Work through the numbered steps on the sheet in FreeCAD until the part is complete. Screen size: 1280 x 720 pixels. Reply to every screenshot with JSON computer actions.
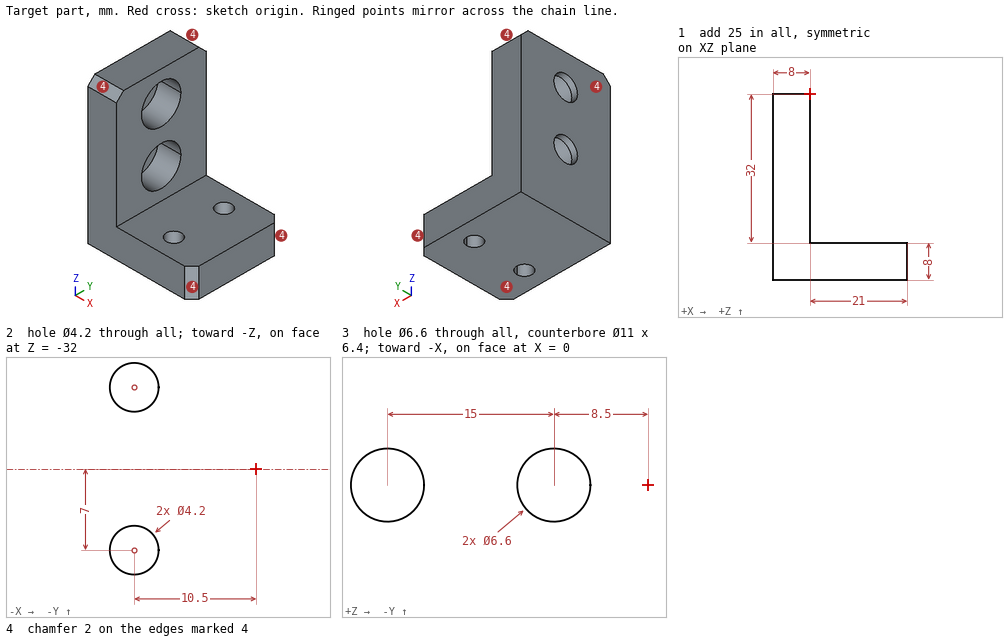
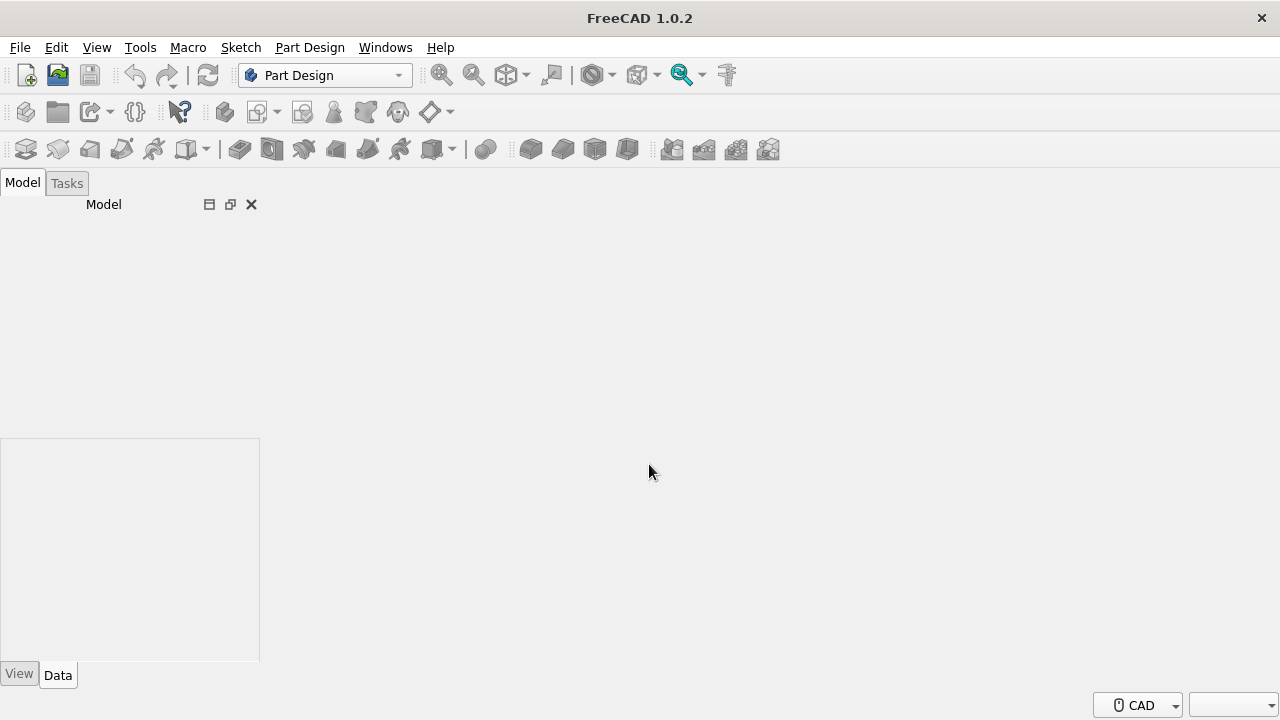
{"action": "left_click", "coordinate": [26, 76]}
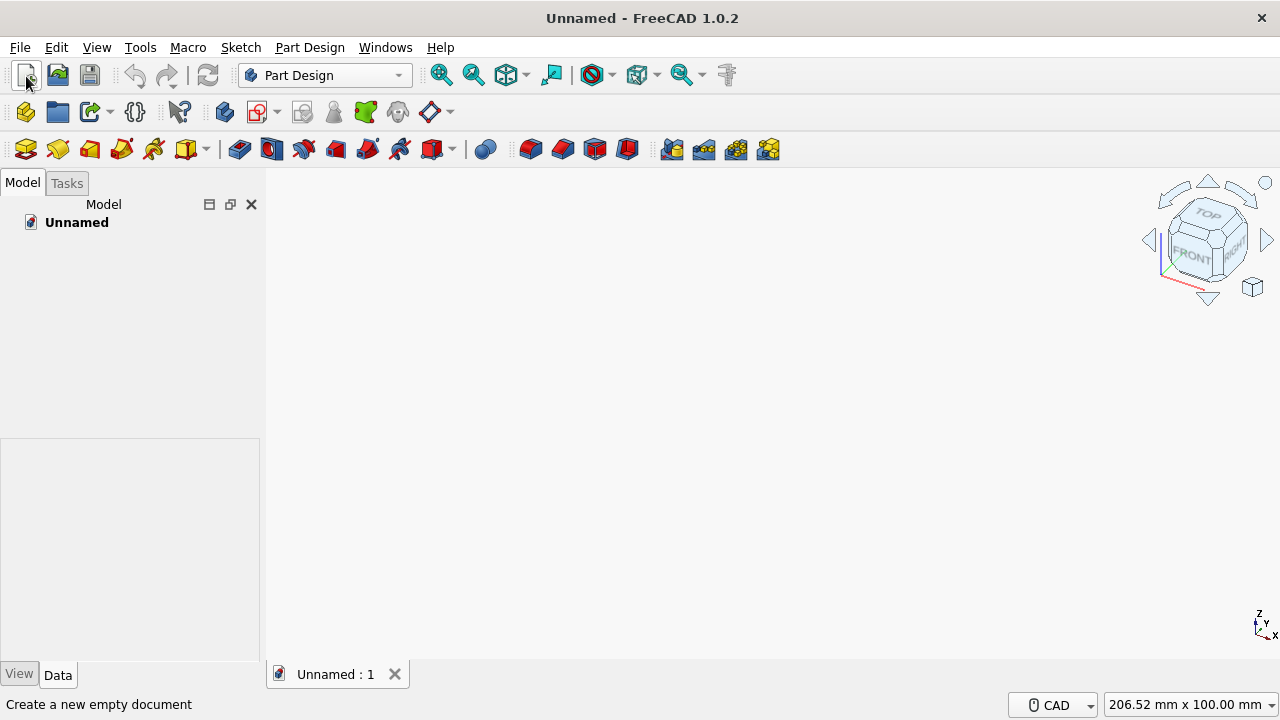
{"action": "left_click", "coordinate": [258, 112]}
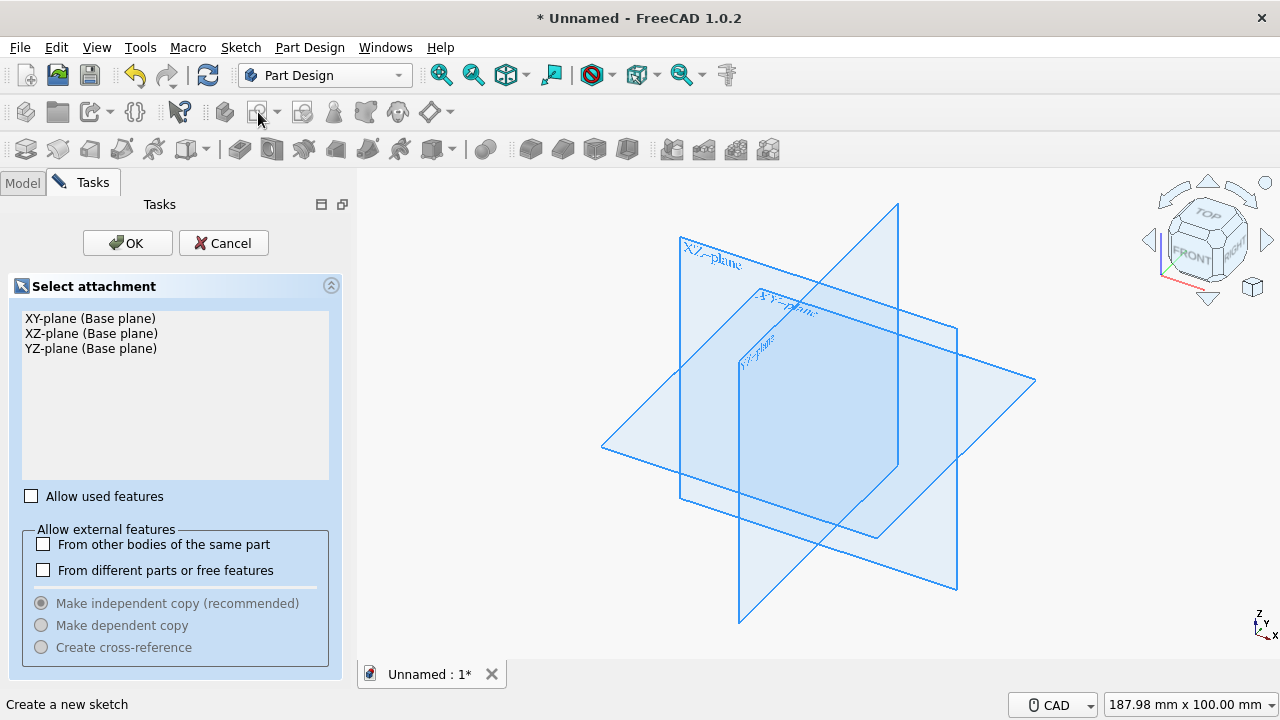
{"action": "left_click", "coordinate": [82, 334]}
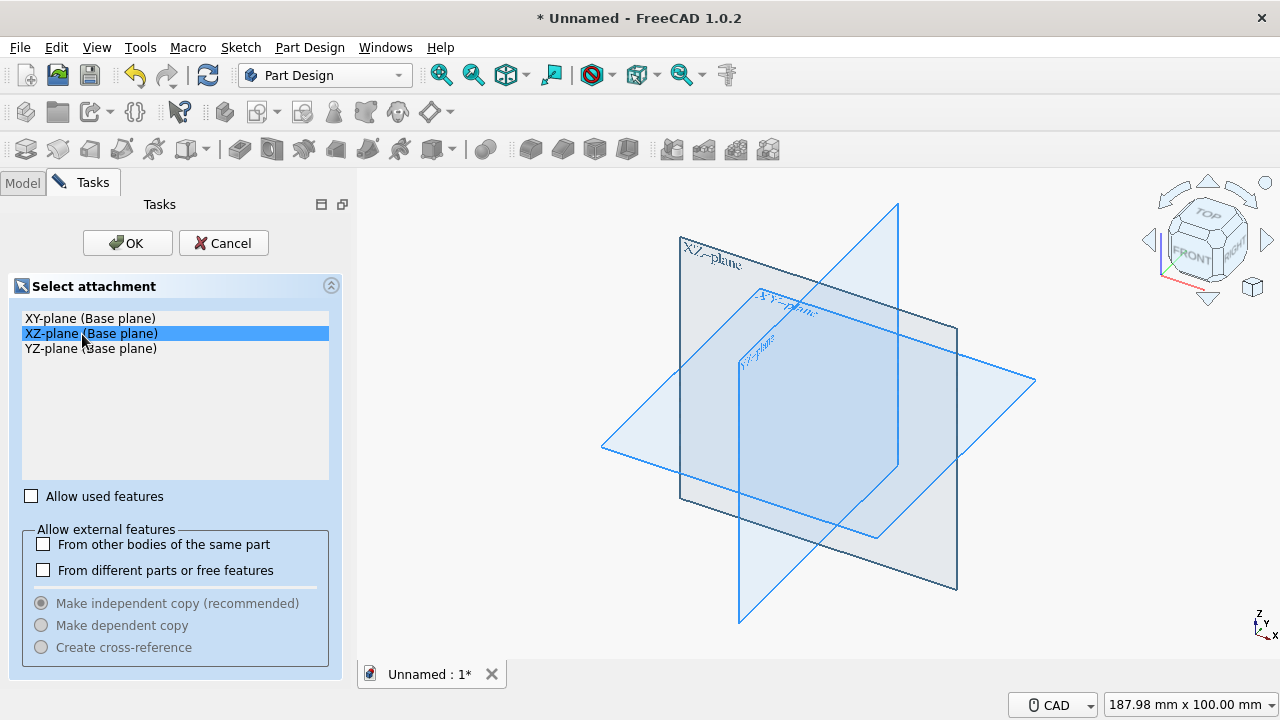
{"action": "left_click", "coordinate": [128, 243]}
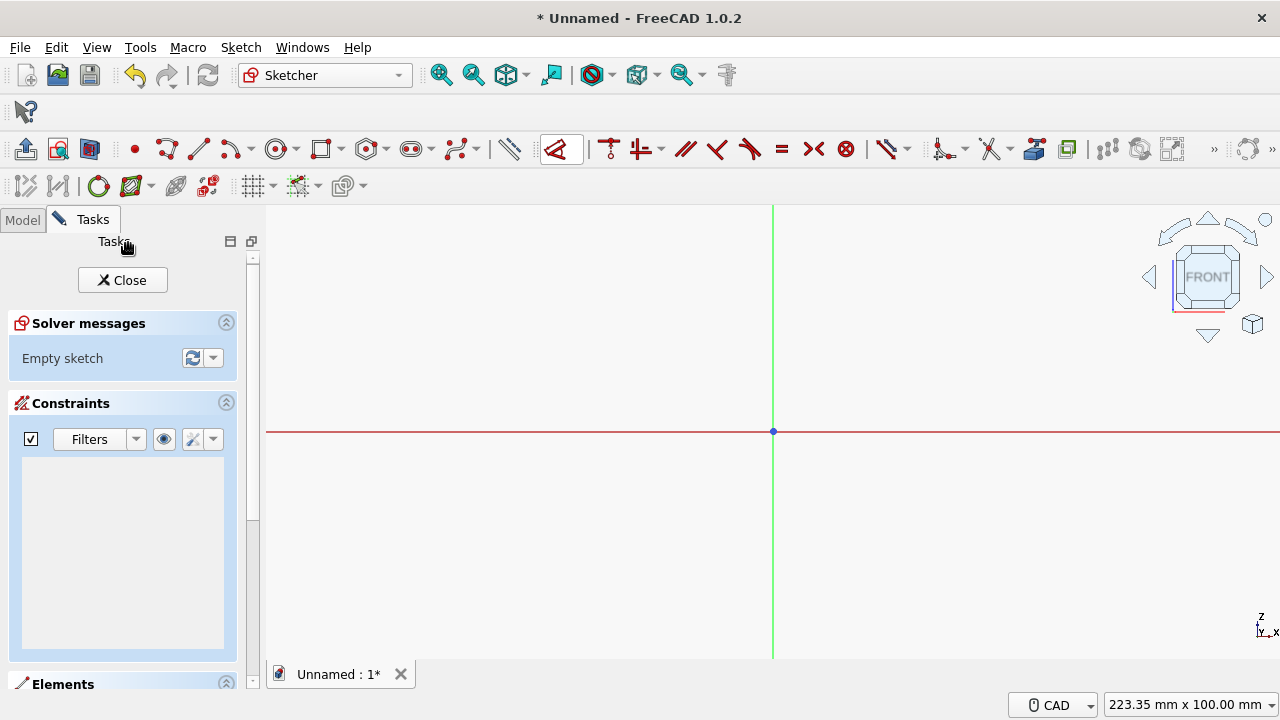
{"action": "scroll", "coordinate": [1002, 631], "scroll_direction": "up", "scroll_amount": 2}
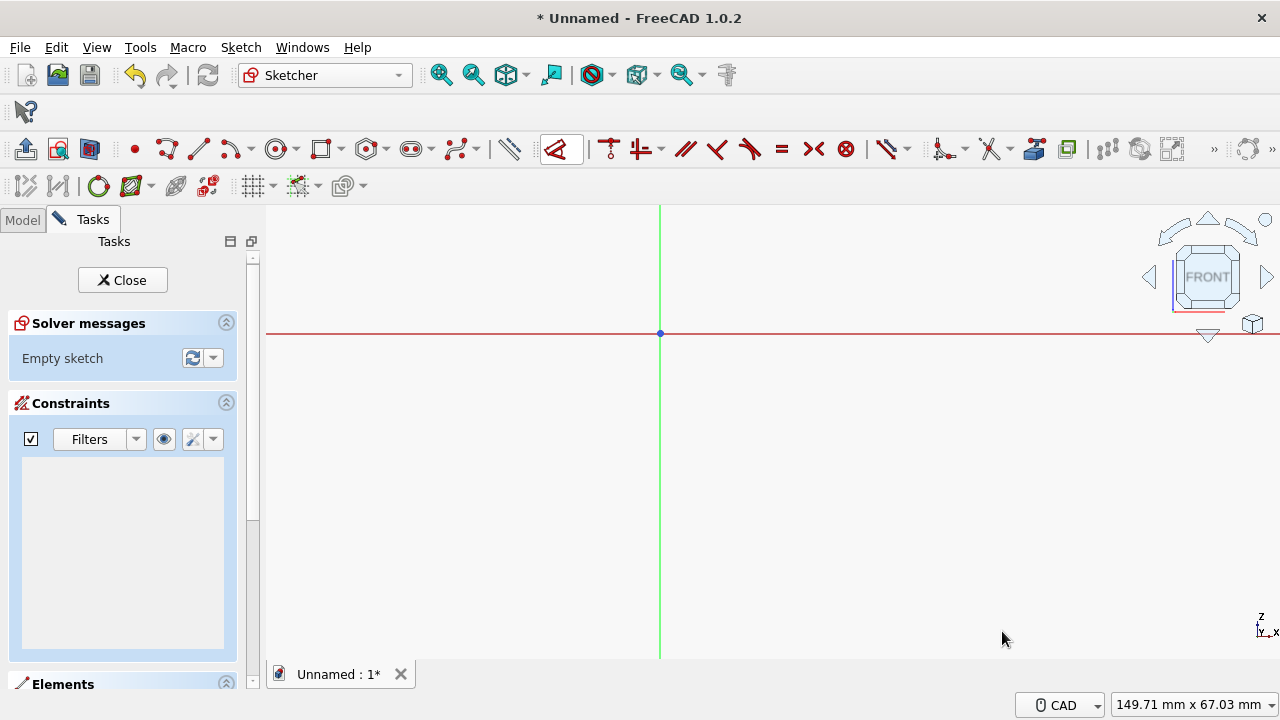
{"action": "left_click", "coordinate": [168, 150]}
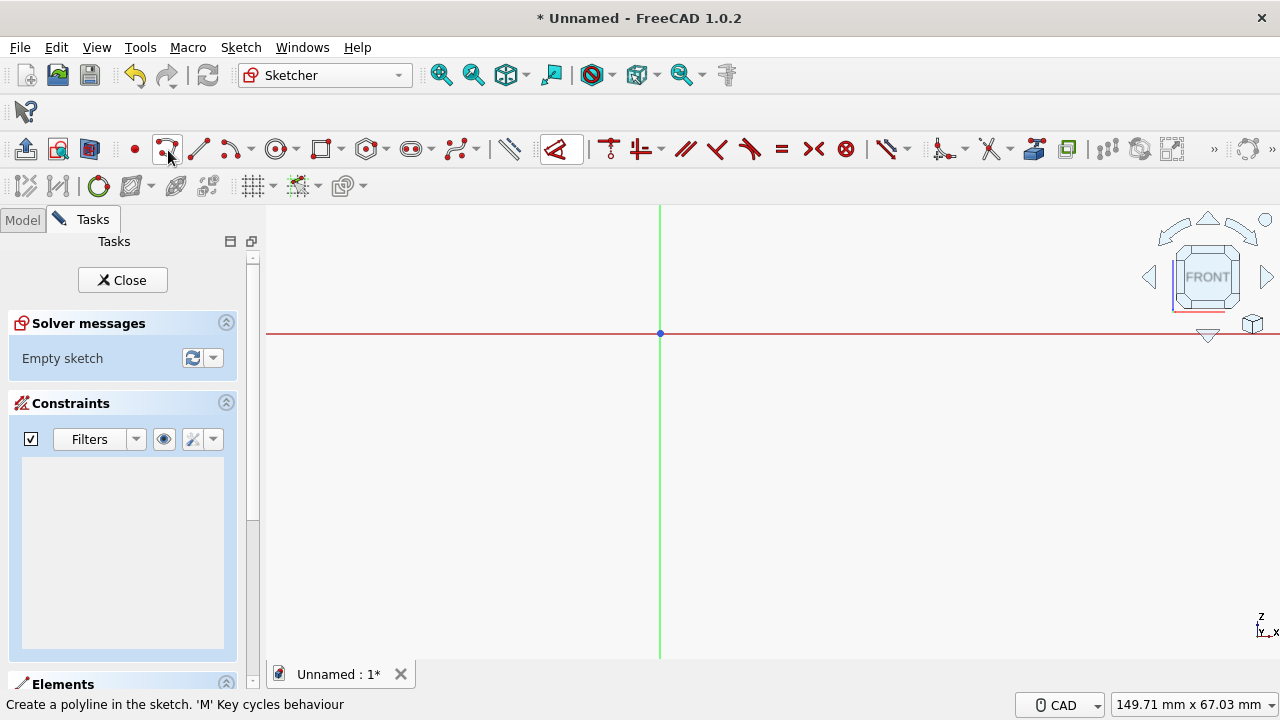
{"action": "left_click", "coordinate": [660, 334]}
{"action": "left_click", "coordinate": [669, 550]}
{"action": "left_click", "coordinate": [802, 550]}
{"action": "left_click", "coordinate": [802, 605]}
{"action": "left_click", "coordinate": [606, 605]}
{"action": "left_click", "coordinate": [606, 343]}
{"action": "left_click", "coordinate": [660, 334]}
{"action": "key", "text": "Escape"}
{"action": "key", "text": "Escape"}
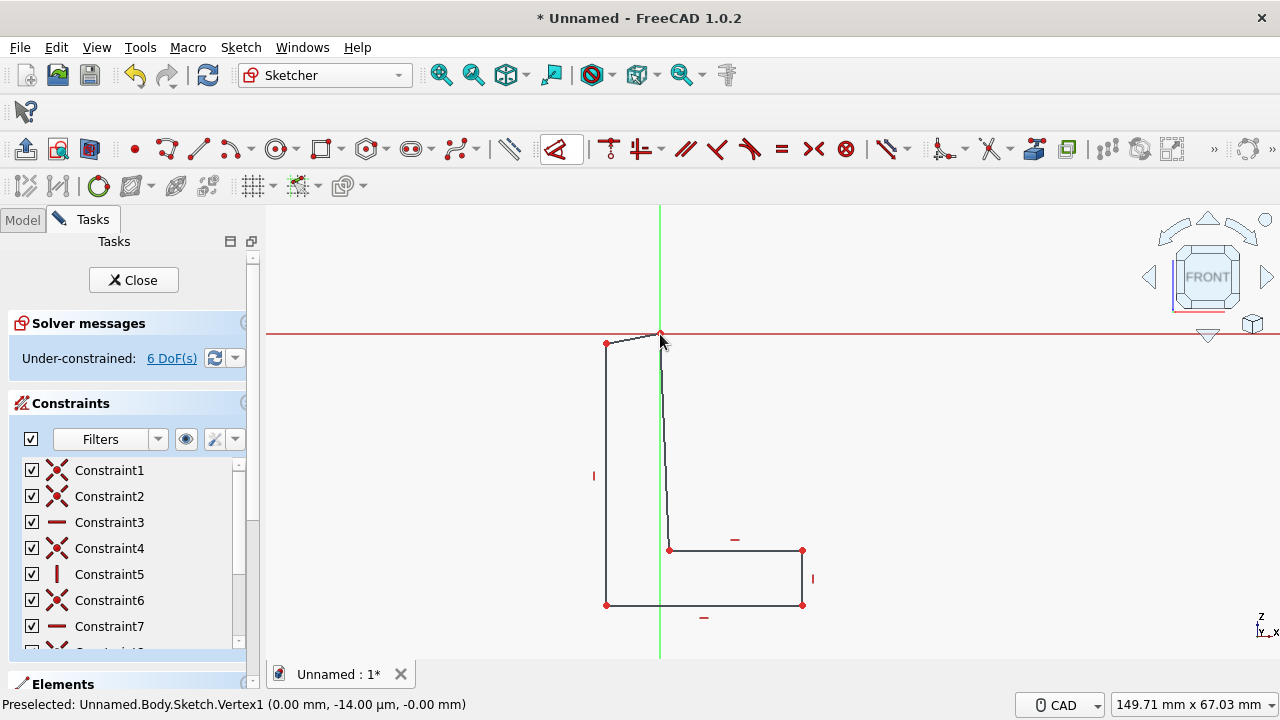
{"action": "left_click", "coordinate": [663, 399]}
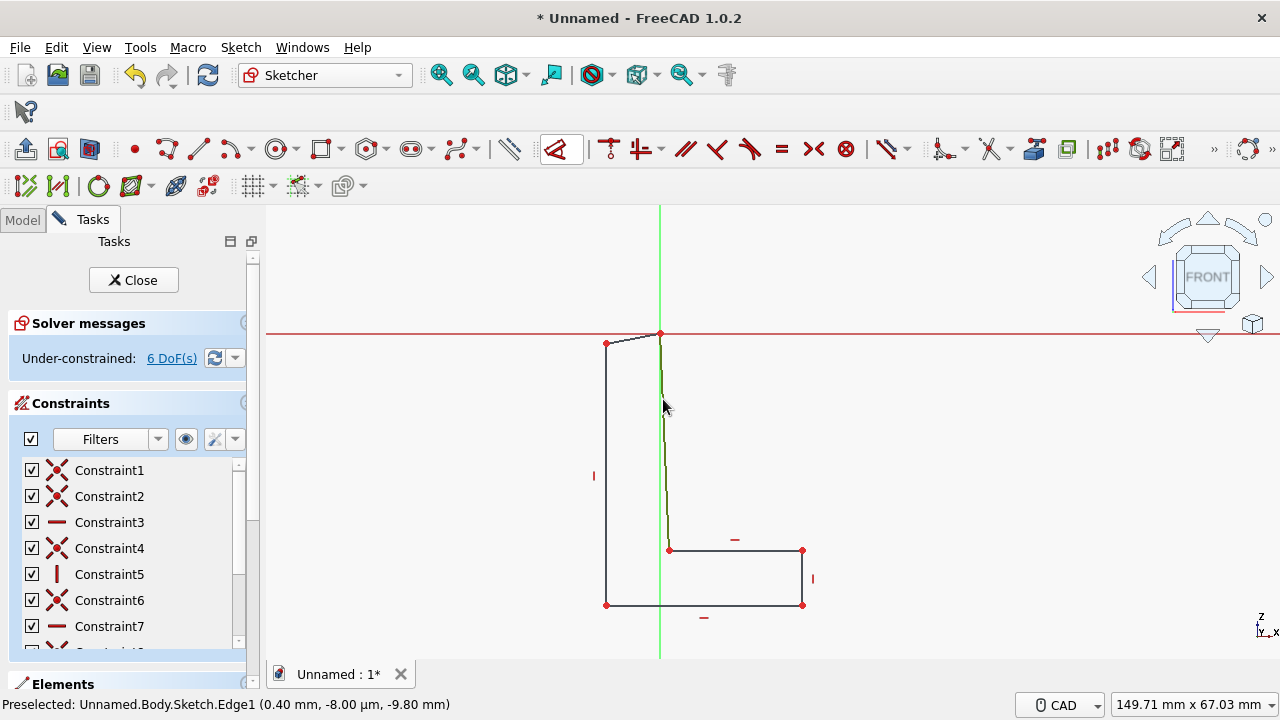
{"action": "left_click", "coordinate": [664, 150]}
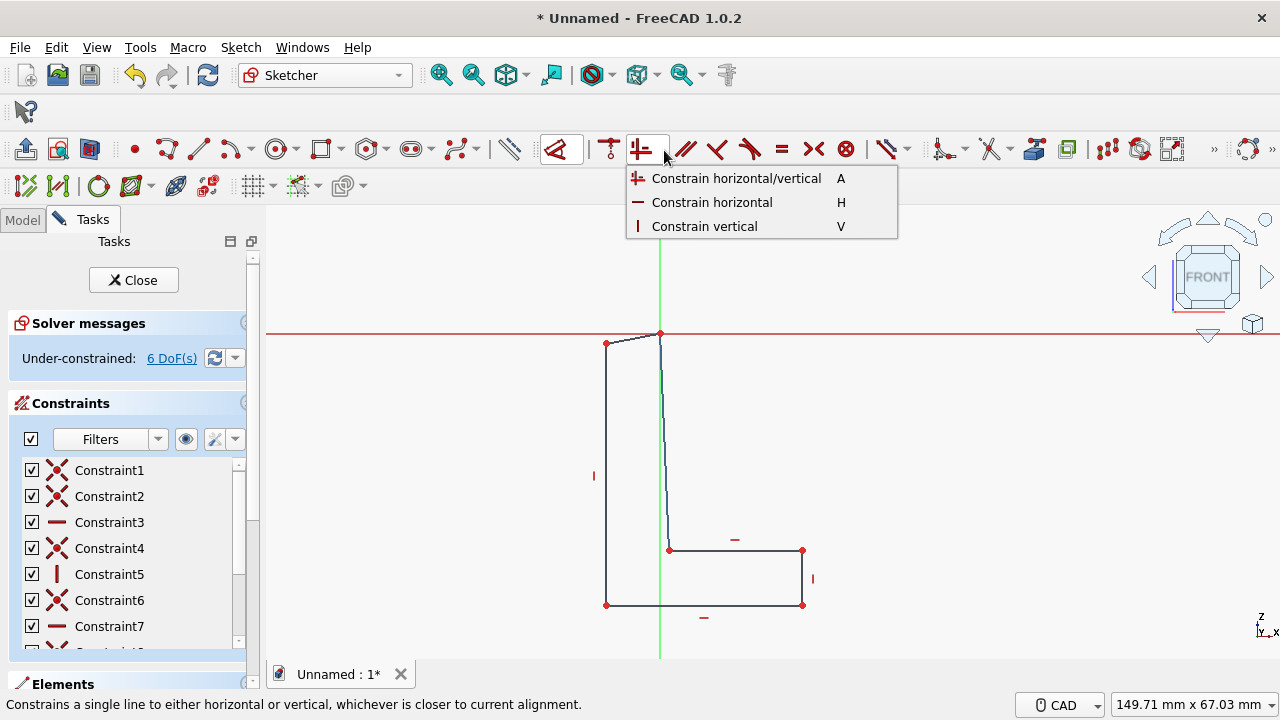
{"action": "left_click", "coordinate": [762, 226]}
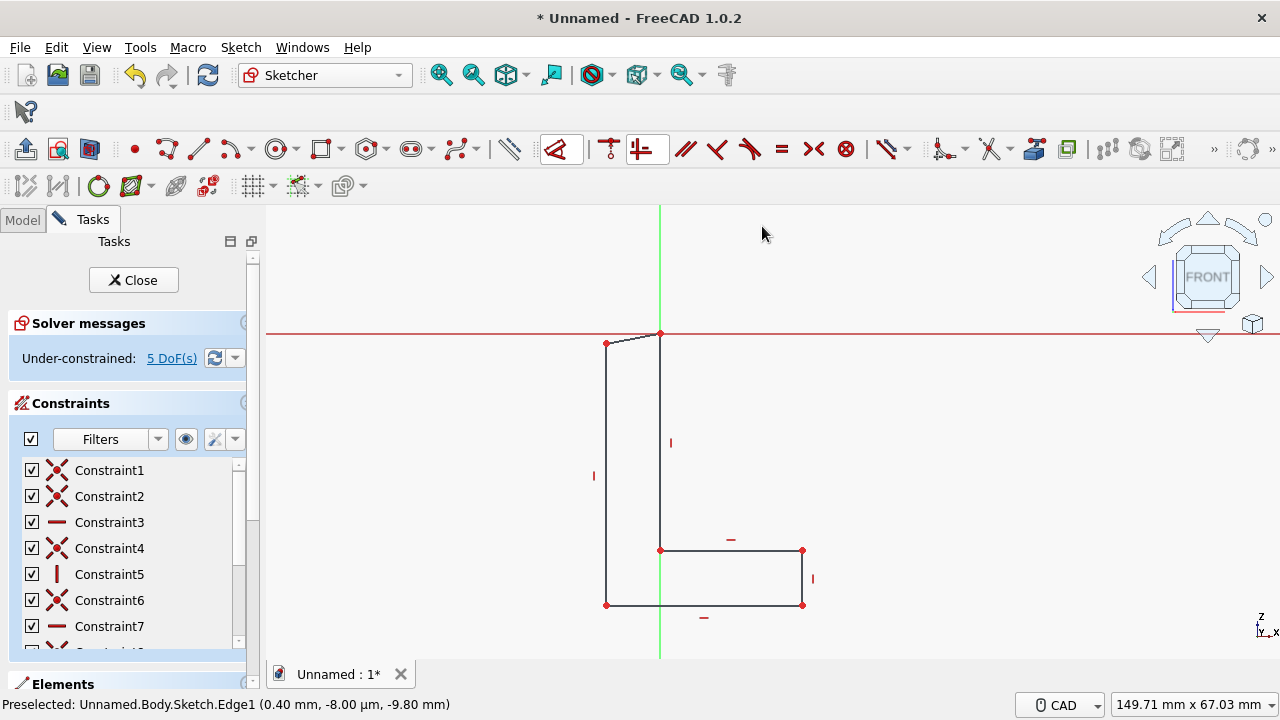
{"action": "left_click", "coordinate": [644, 337]}